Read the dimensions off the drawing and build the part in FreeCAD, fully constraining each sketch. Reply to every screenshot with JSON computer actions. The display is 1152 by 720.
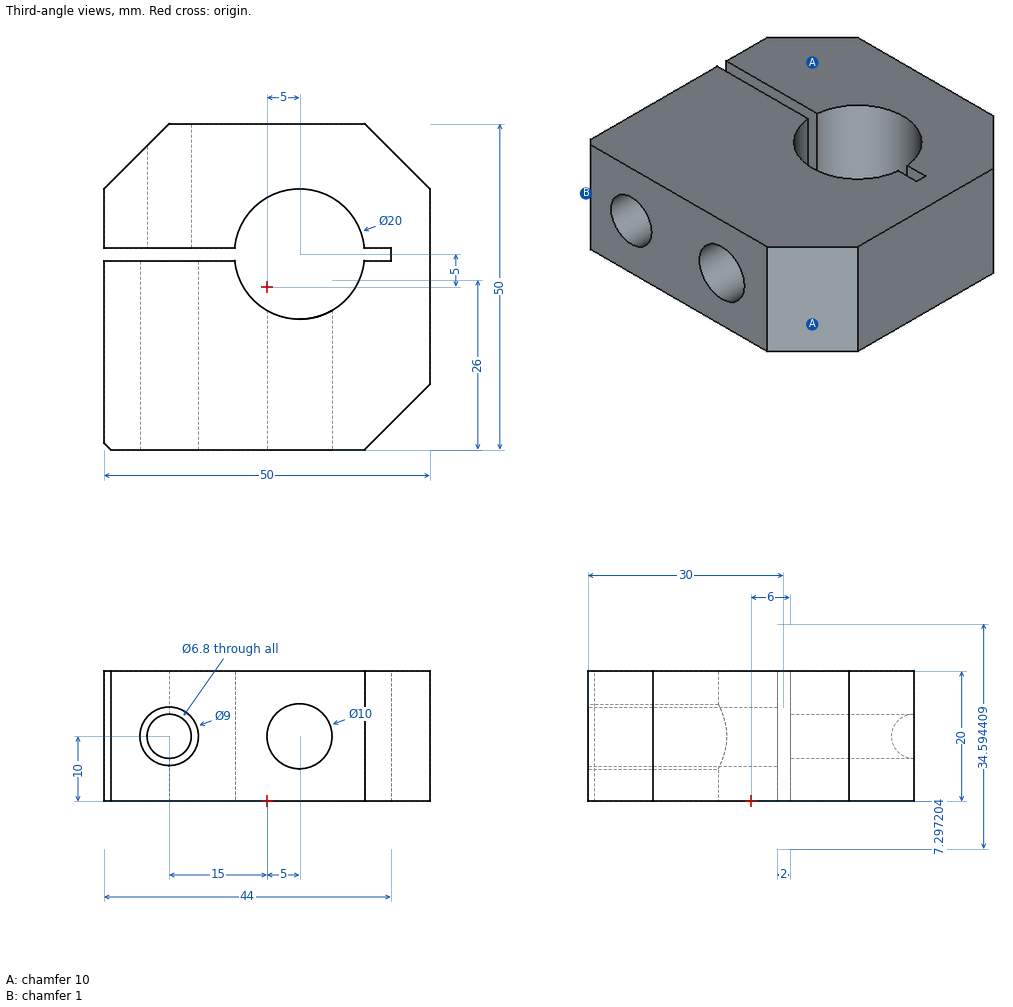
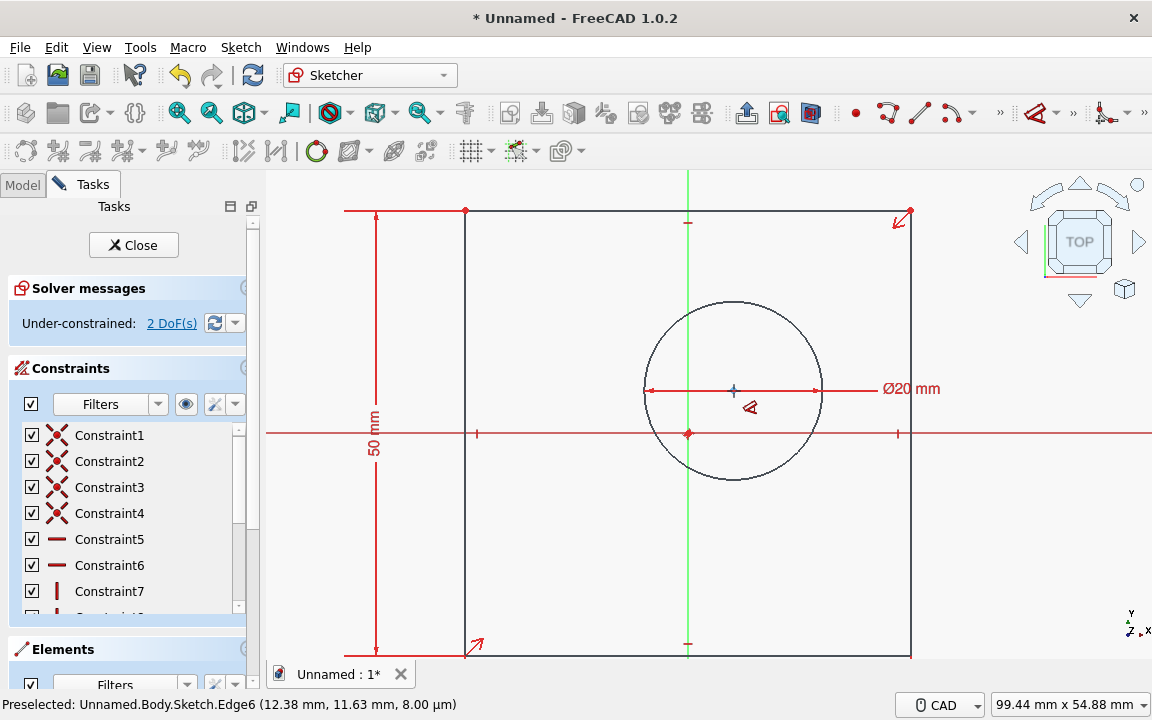
{"action": "left_click", "coordinate": [733, 391]}
{"action": "left_click", "coordinate": [711, 357]}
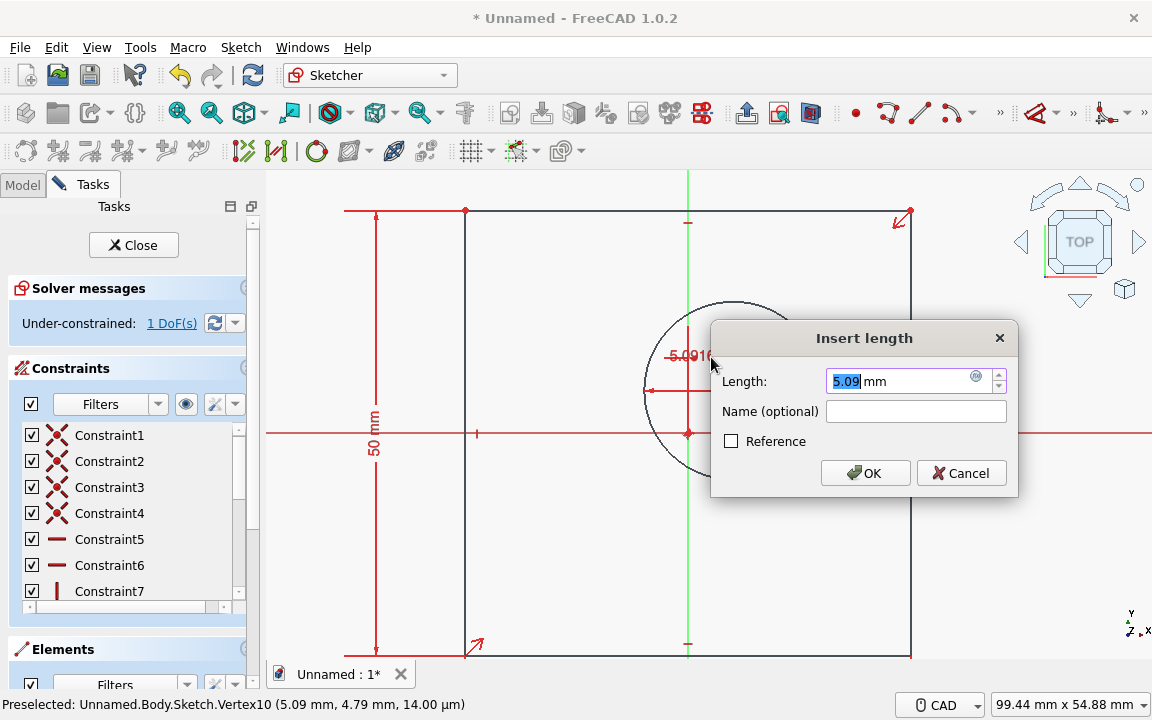
{"action": "type", "text": "5"}
{"action": "key", "text": "Return"}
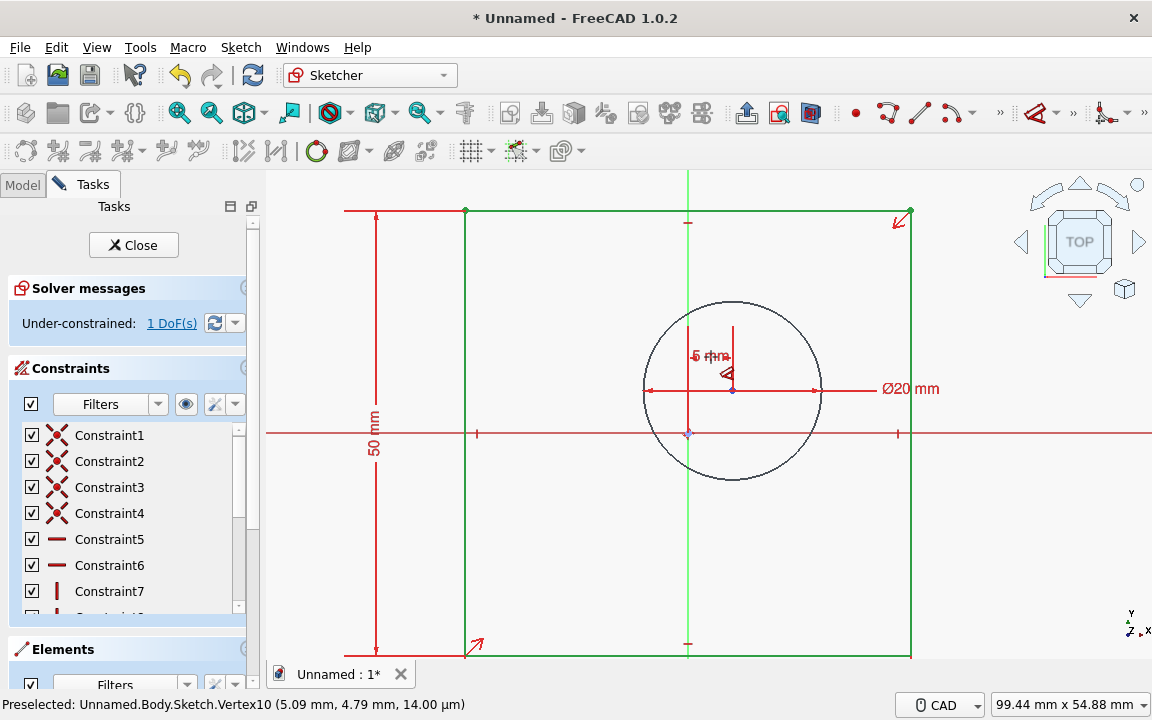
{"action": "left_click", "coordinate": [733, 391]}
{"action": "left_click", "coordinate": [767, 412]}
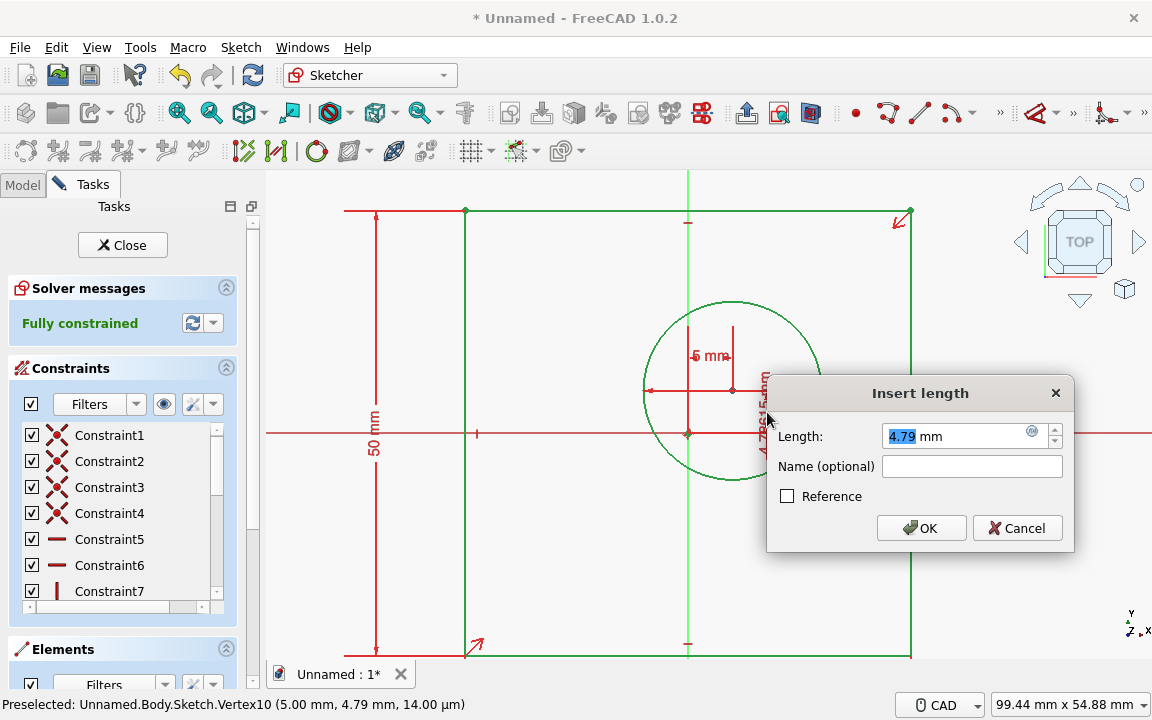
{"action": "type", "text": "5"}
{"action": "key", "text": "Return"}
{"action": "key", "text": "Escape"}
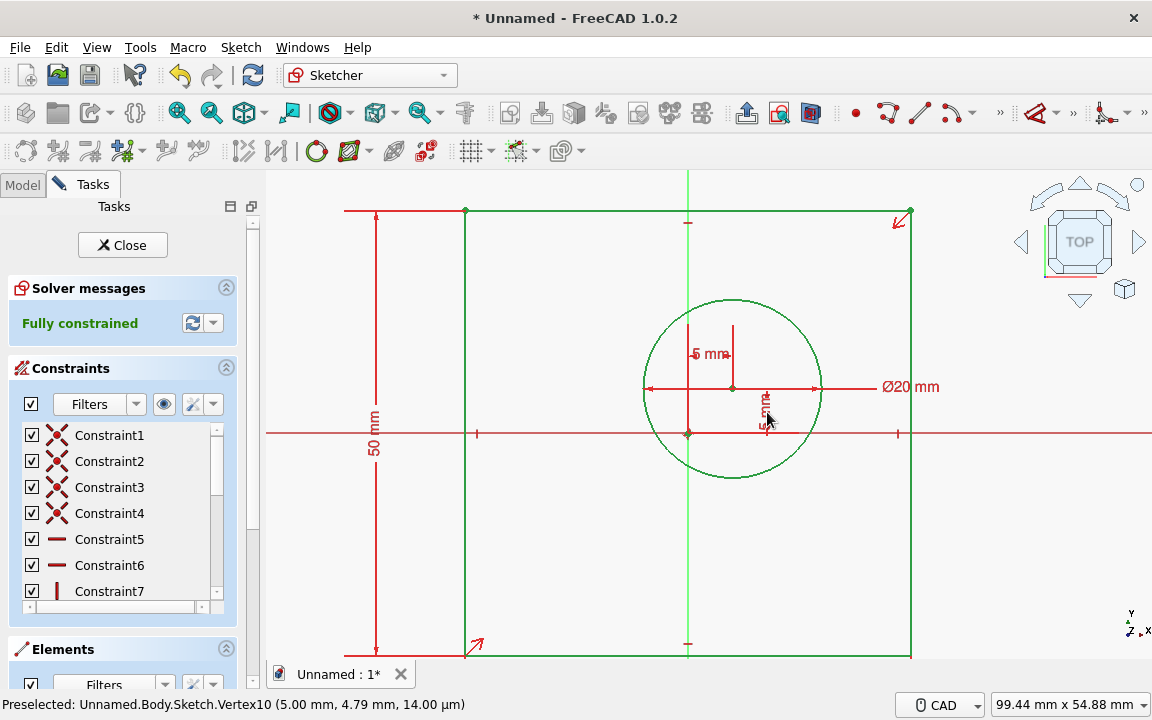
{"action": "left_click", "coordinate": [123, 245]}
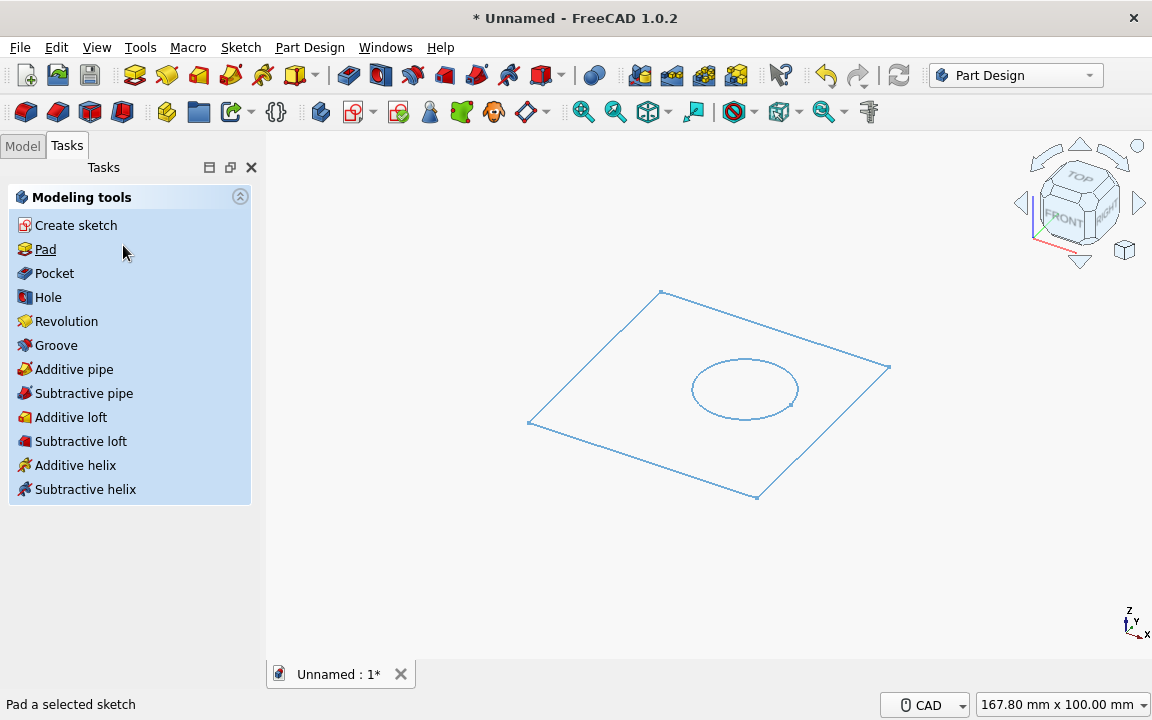
{"action": "left_click", "coordinate": [136, 76]}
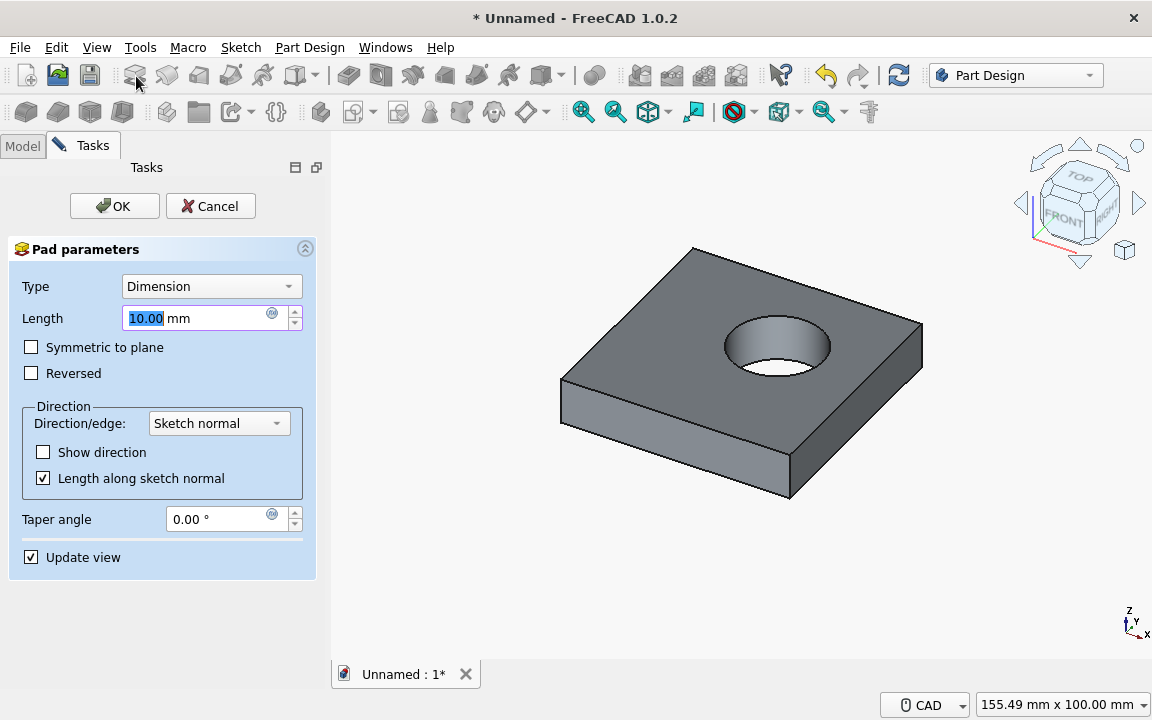
{"action": "type", "text": "20"}
{"action": "key", "text": "Tab"}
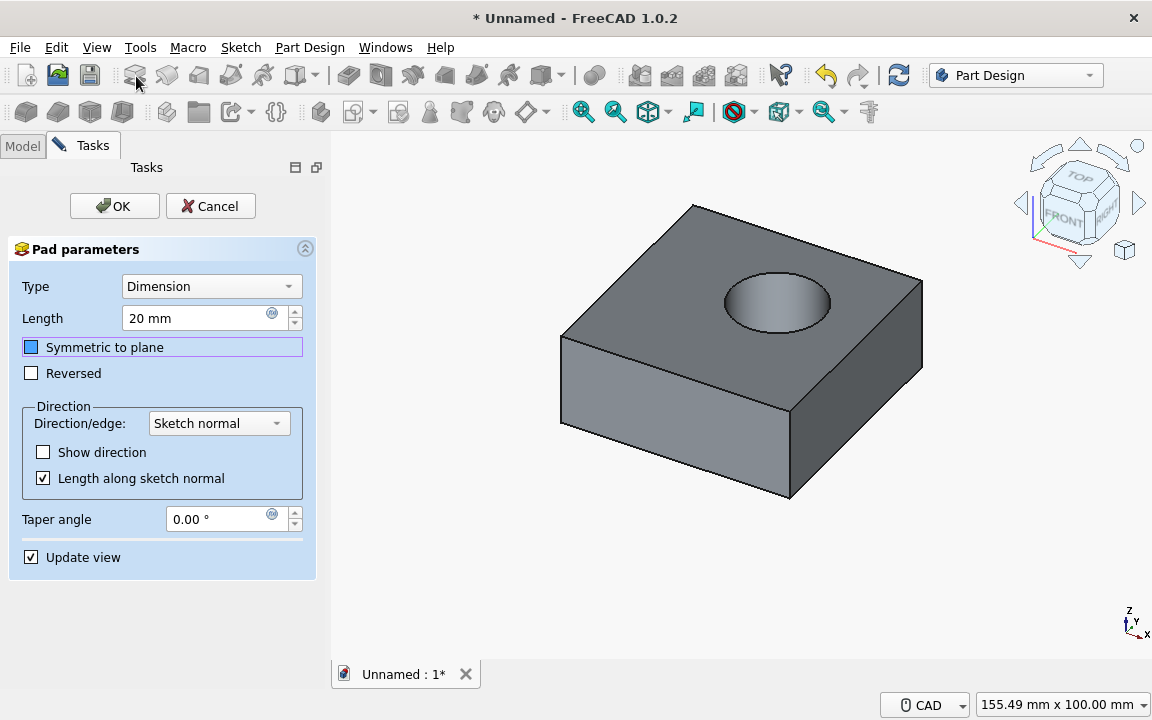
{"action": "left_click", "coordinate": [115, 206]}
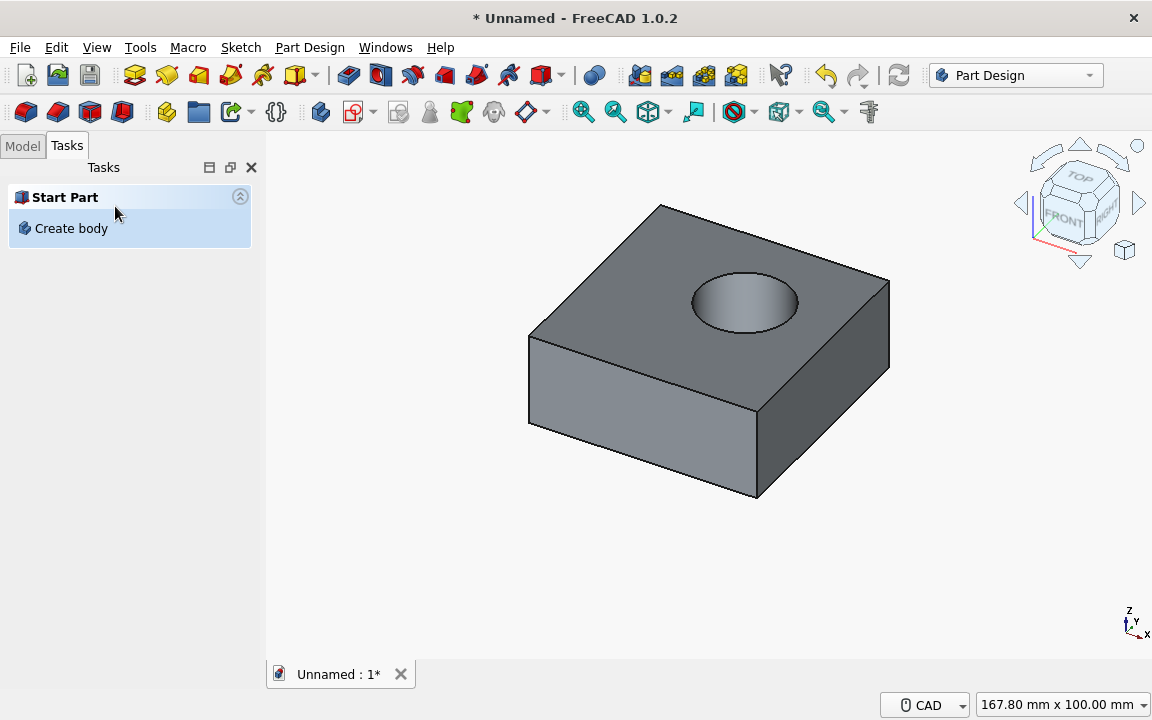
{"action": "left_click", "coordinate": [757, 454]}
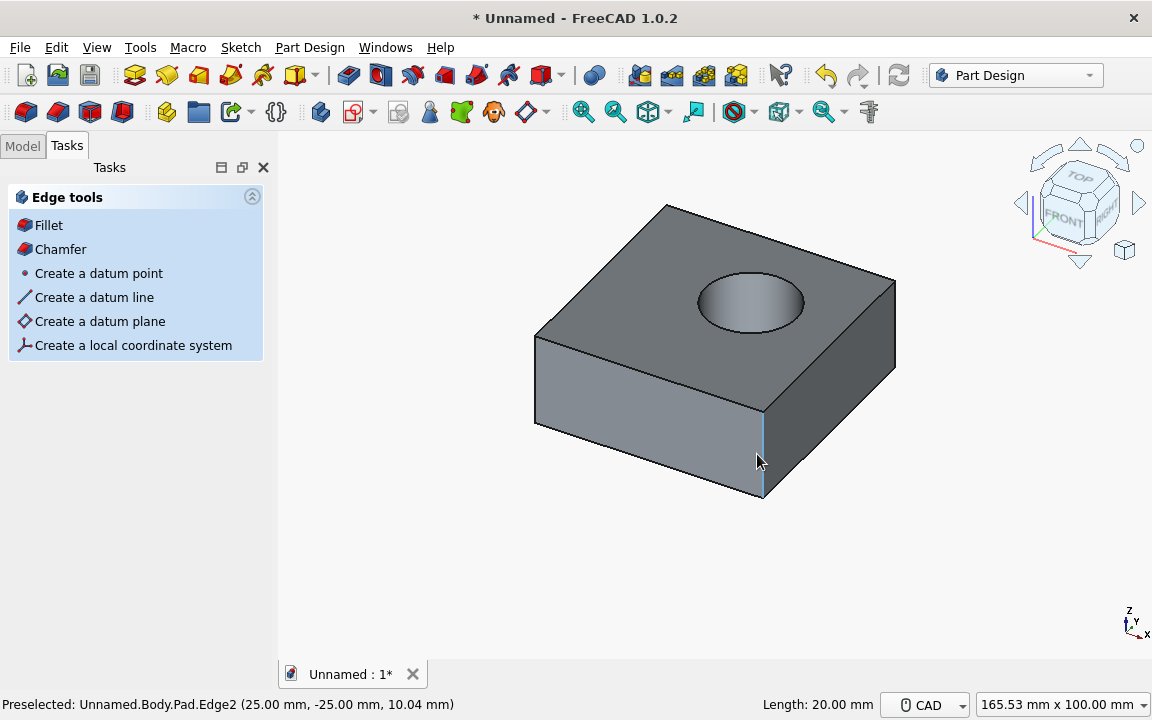
{"action": "key", "text": "0"}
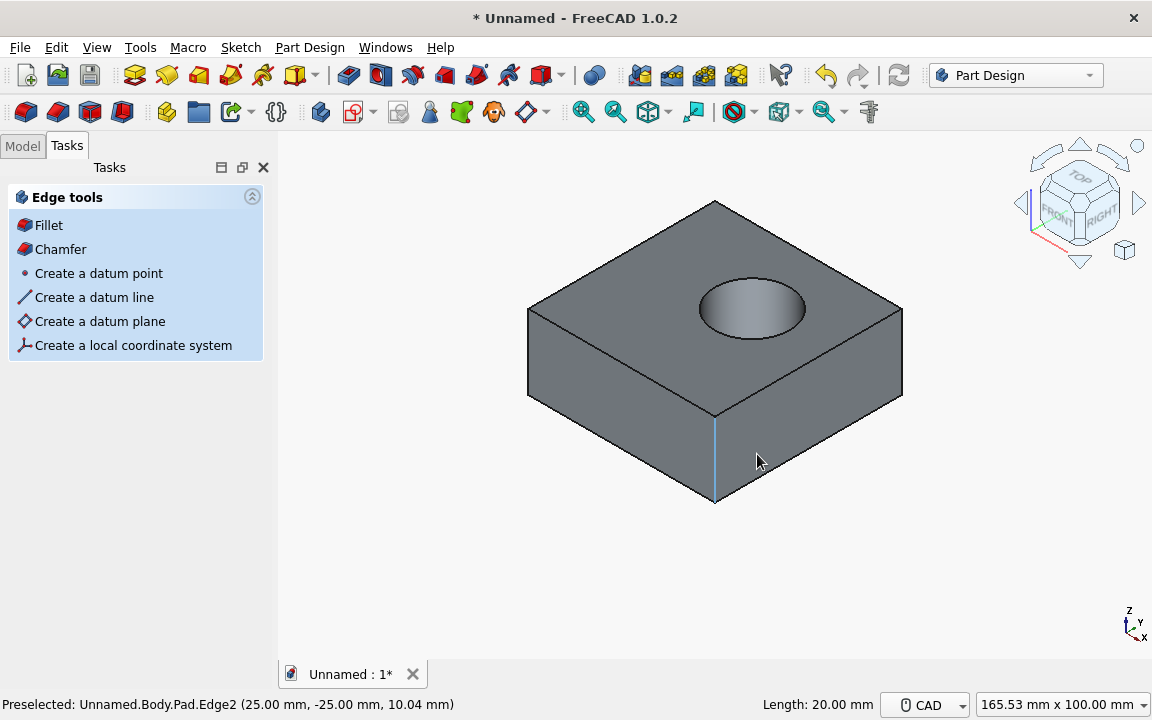
{"action": "key", "text": "2"}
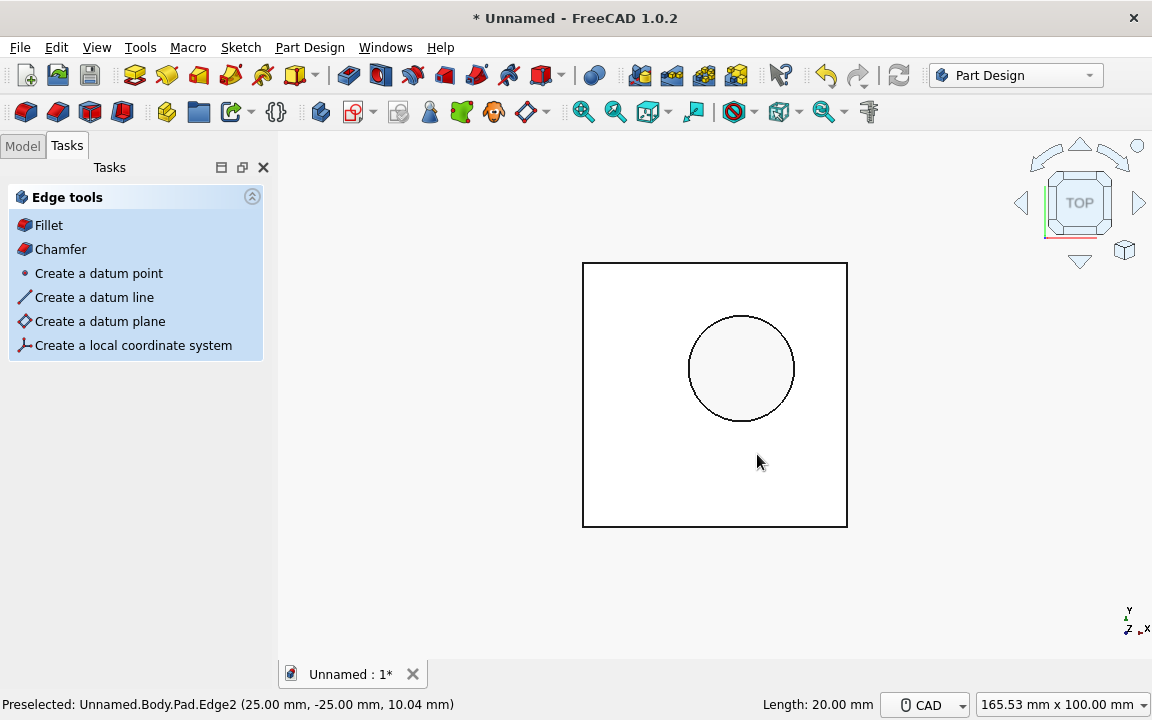
{"action": "key", "text": "1"}